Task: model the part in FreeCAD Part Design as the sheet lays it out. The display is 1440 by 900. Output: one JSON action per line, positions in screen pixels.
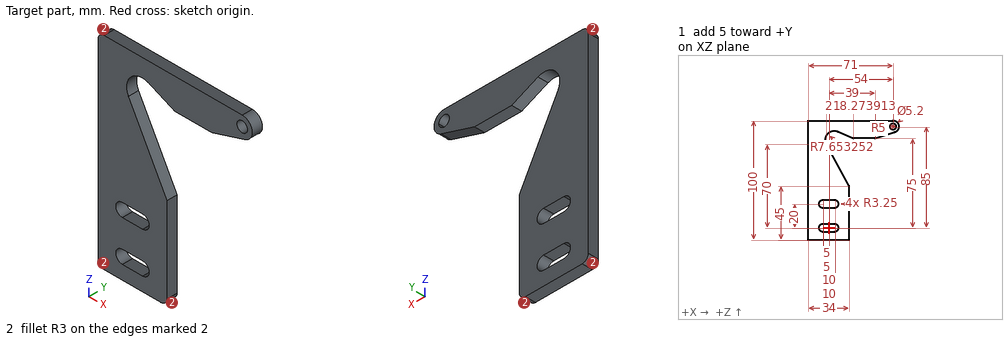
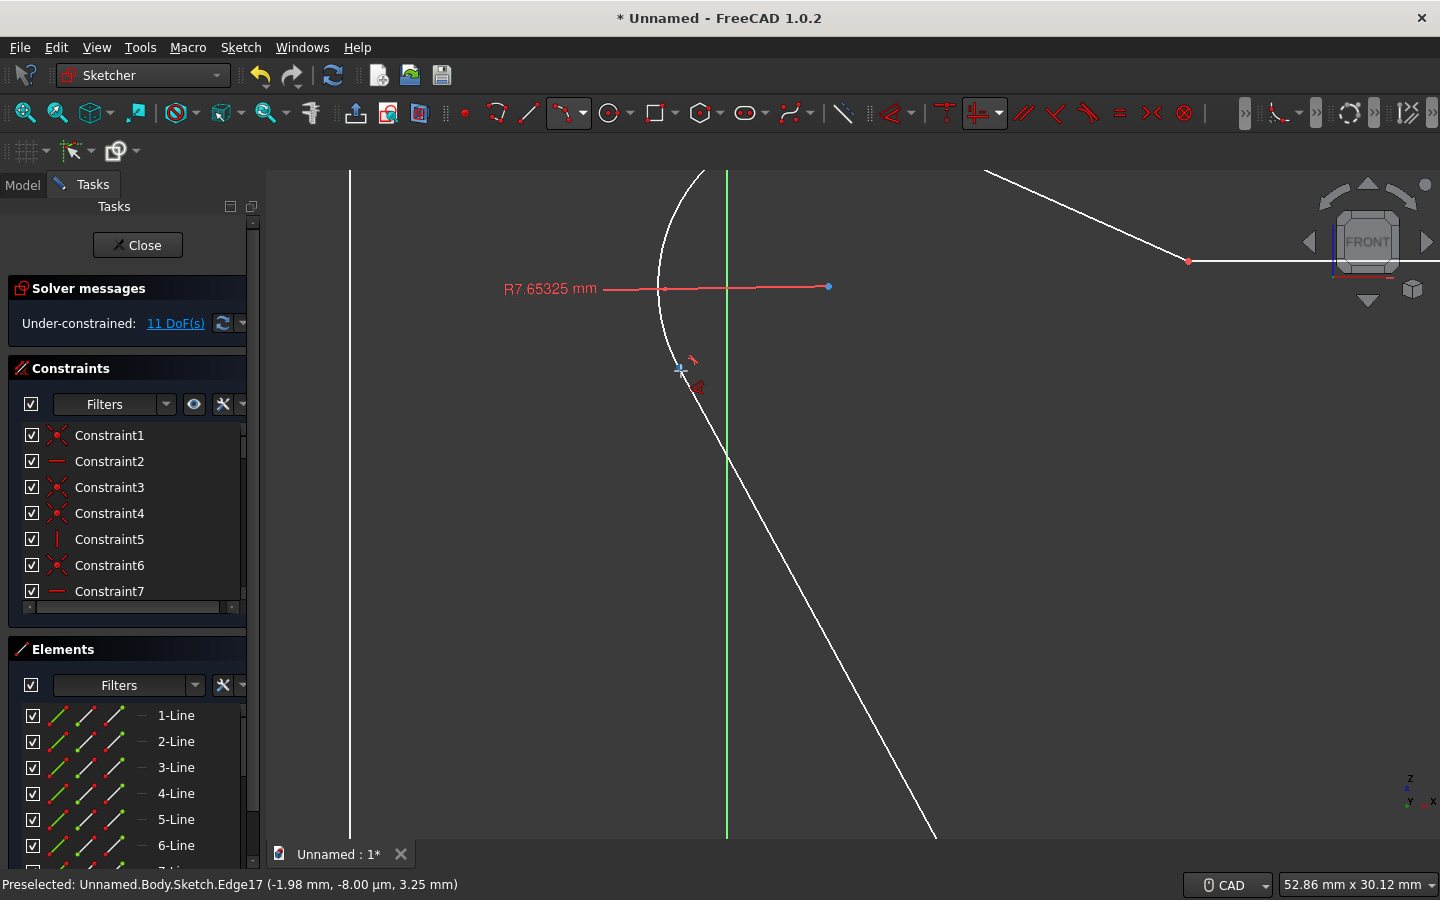
{"action": "left_click", "coordinate": [679, 368]}
{"action": "left_click", "coordinate": [703, 334]}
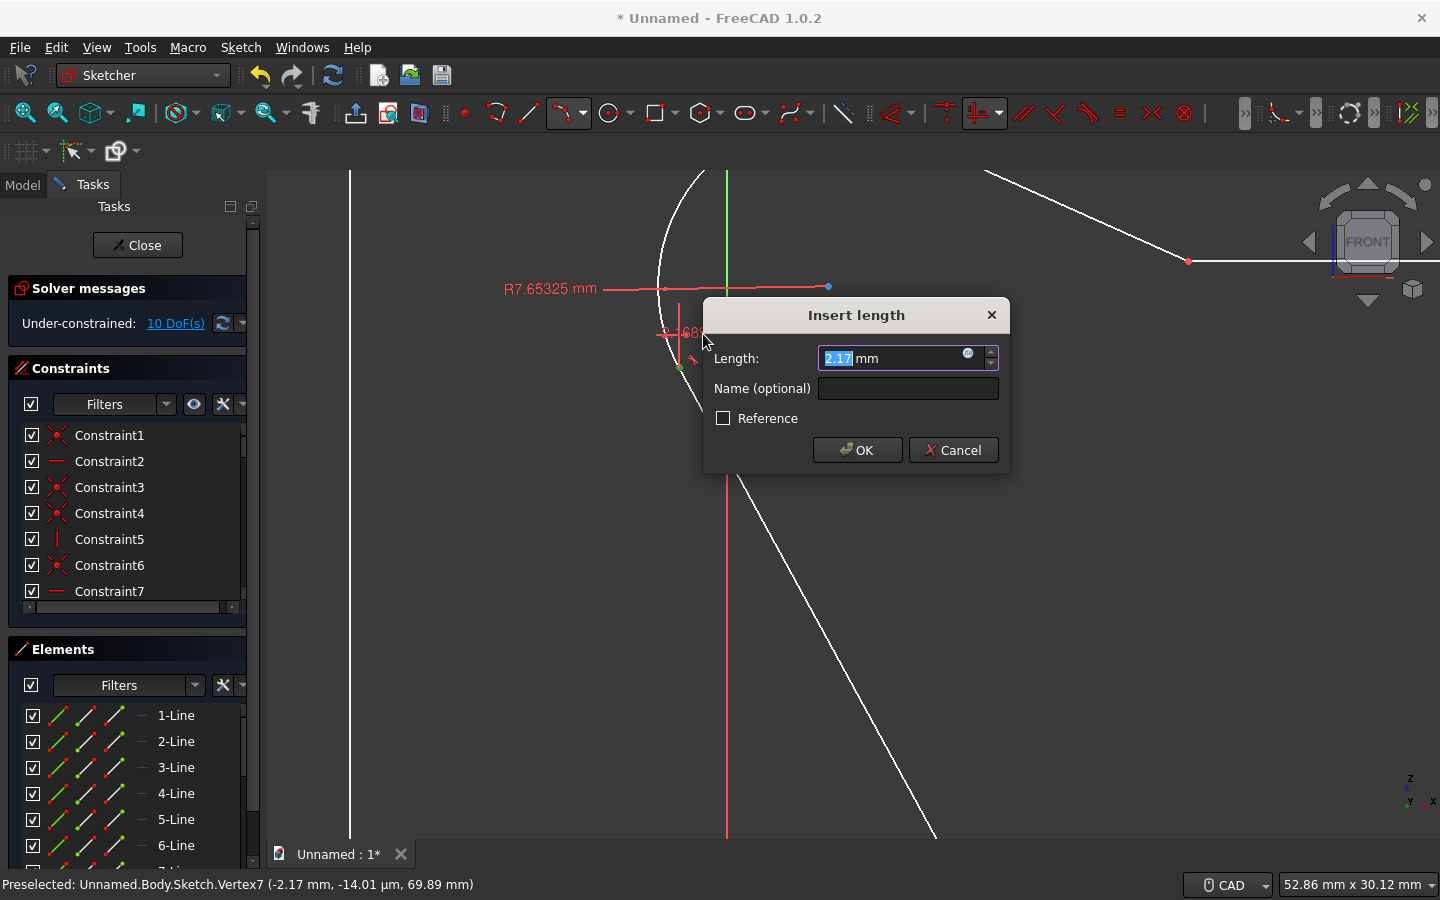
{"action": "type", "text": "2"}
{"action": "key", "text": "Return"}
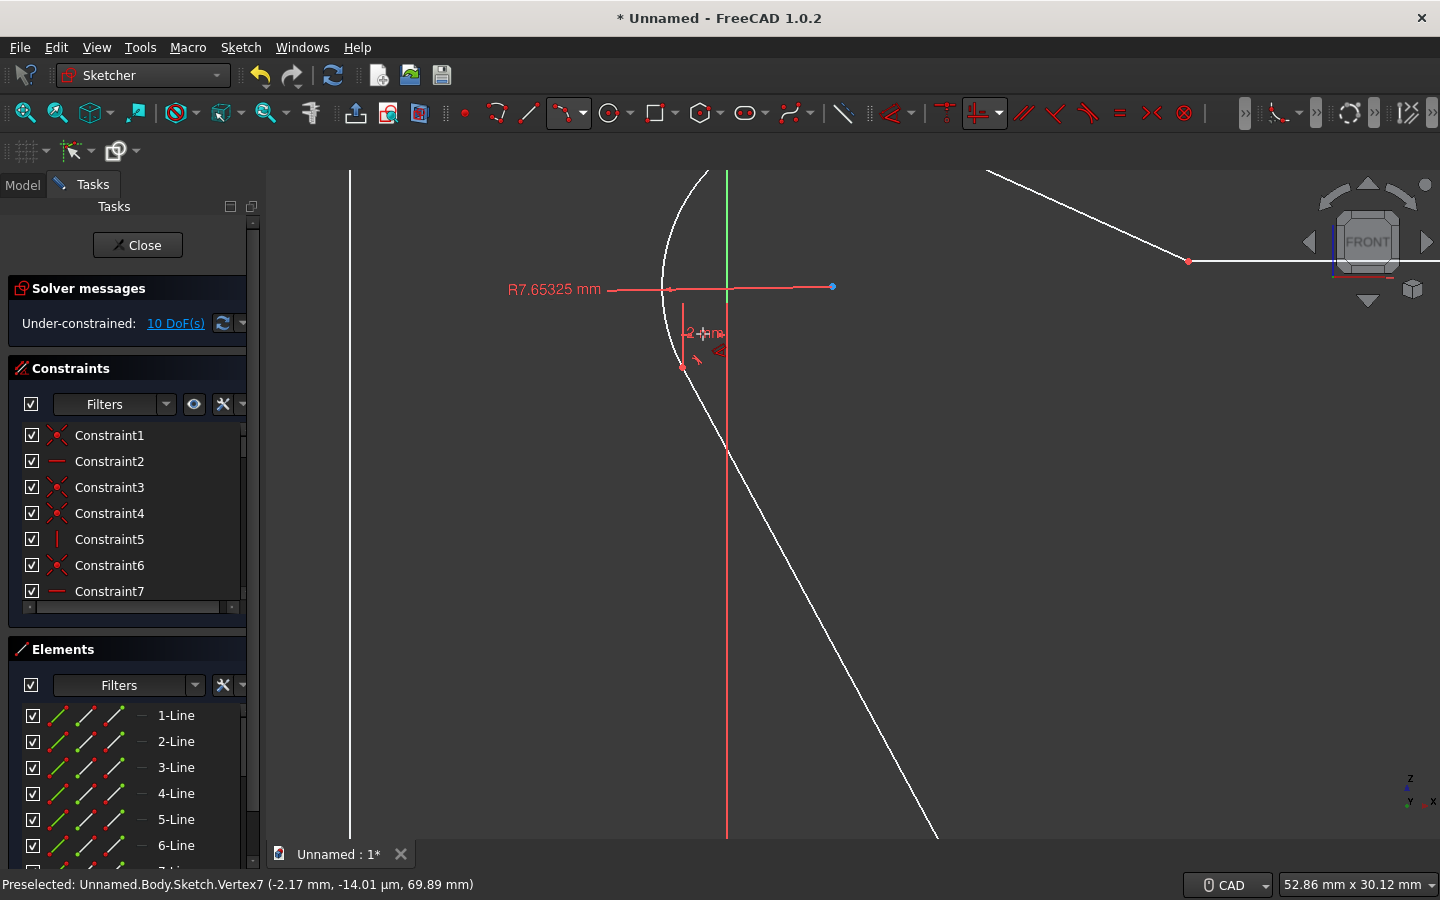
{"action": "scroll", "coordinate": [681, 371], "scroll_direction": "down", "scroll_amount": 8}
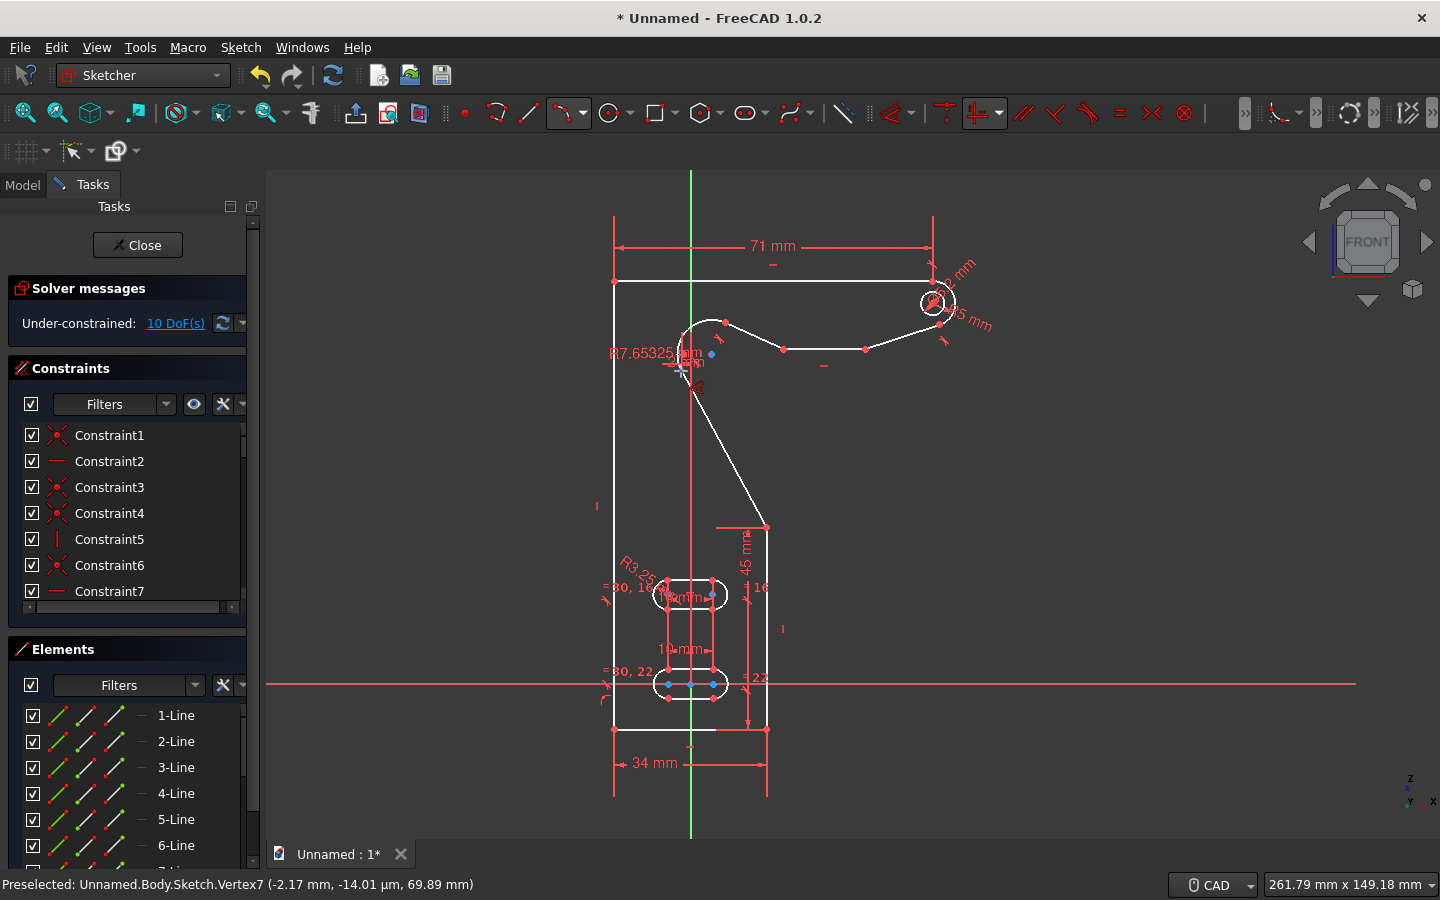
{"action": "scroll", "coordinate": [668, 580], "scroll_direction": "up", "scroll_amount": 3}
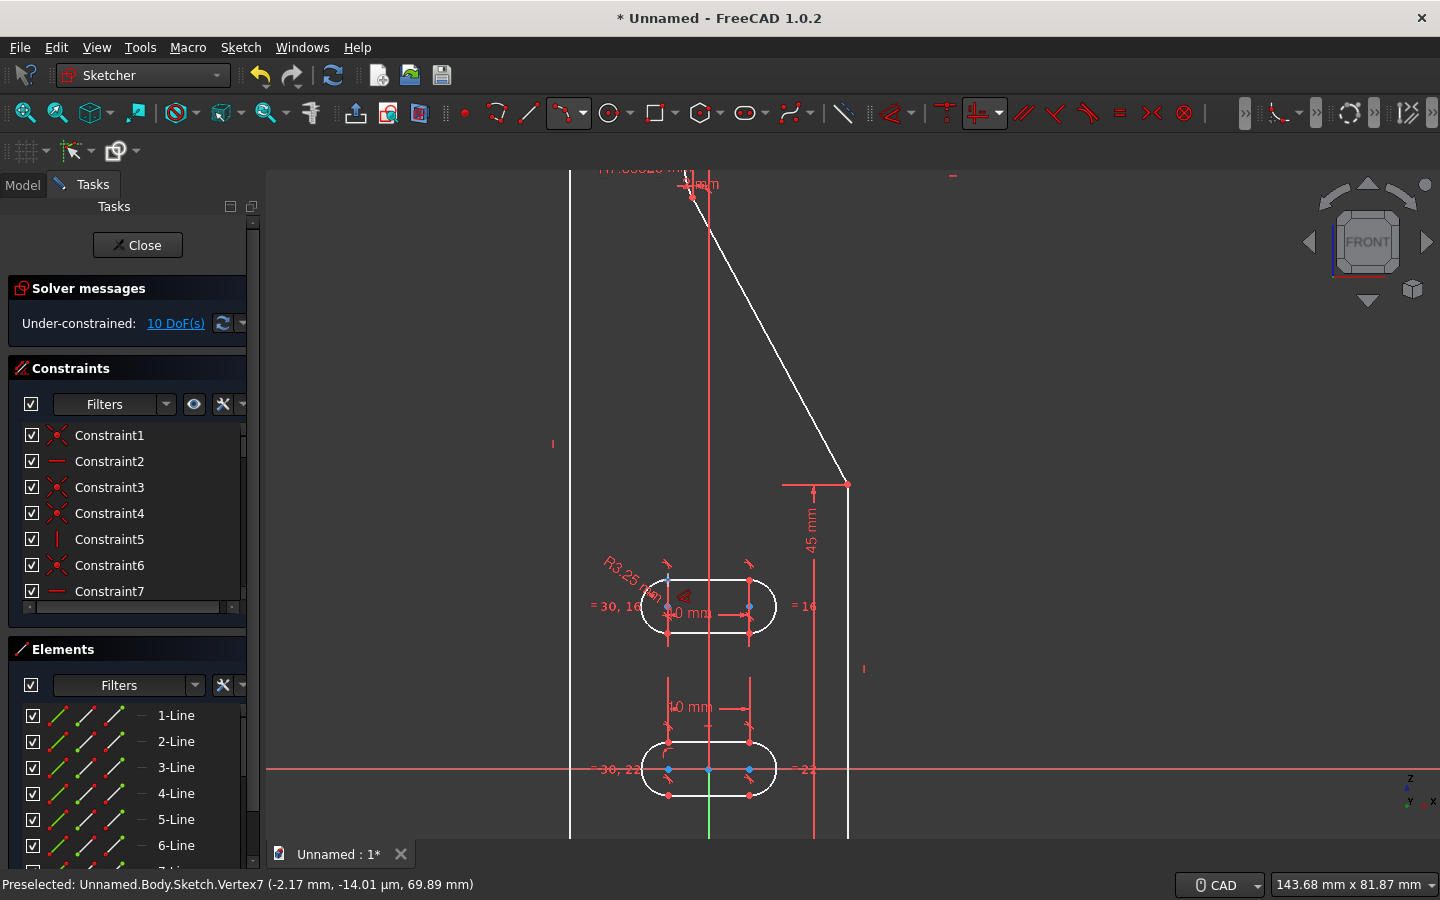
{"action": "left_click", "coordinate": [668, 580]}
{"action": "left_click", "coordinate": [688, 546]}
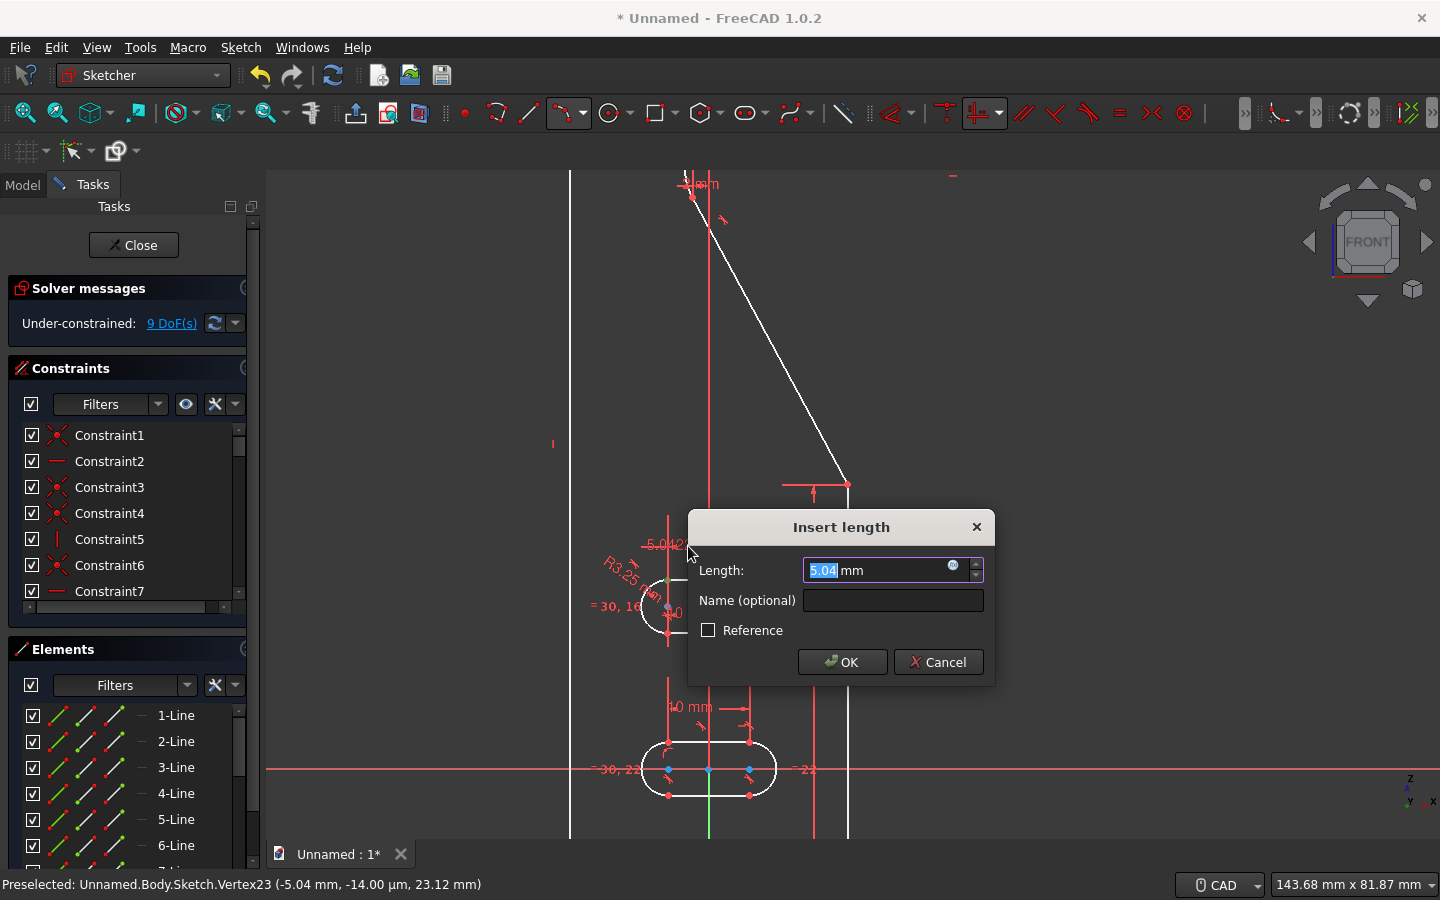
{"action": "type", "text": "5"}
{"action": "key", "text": "Return"}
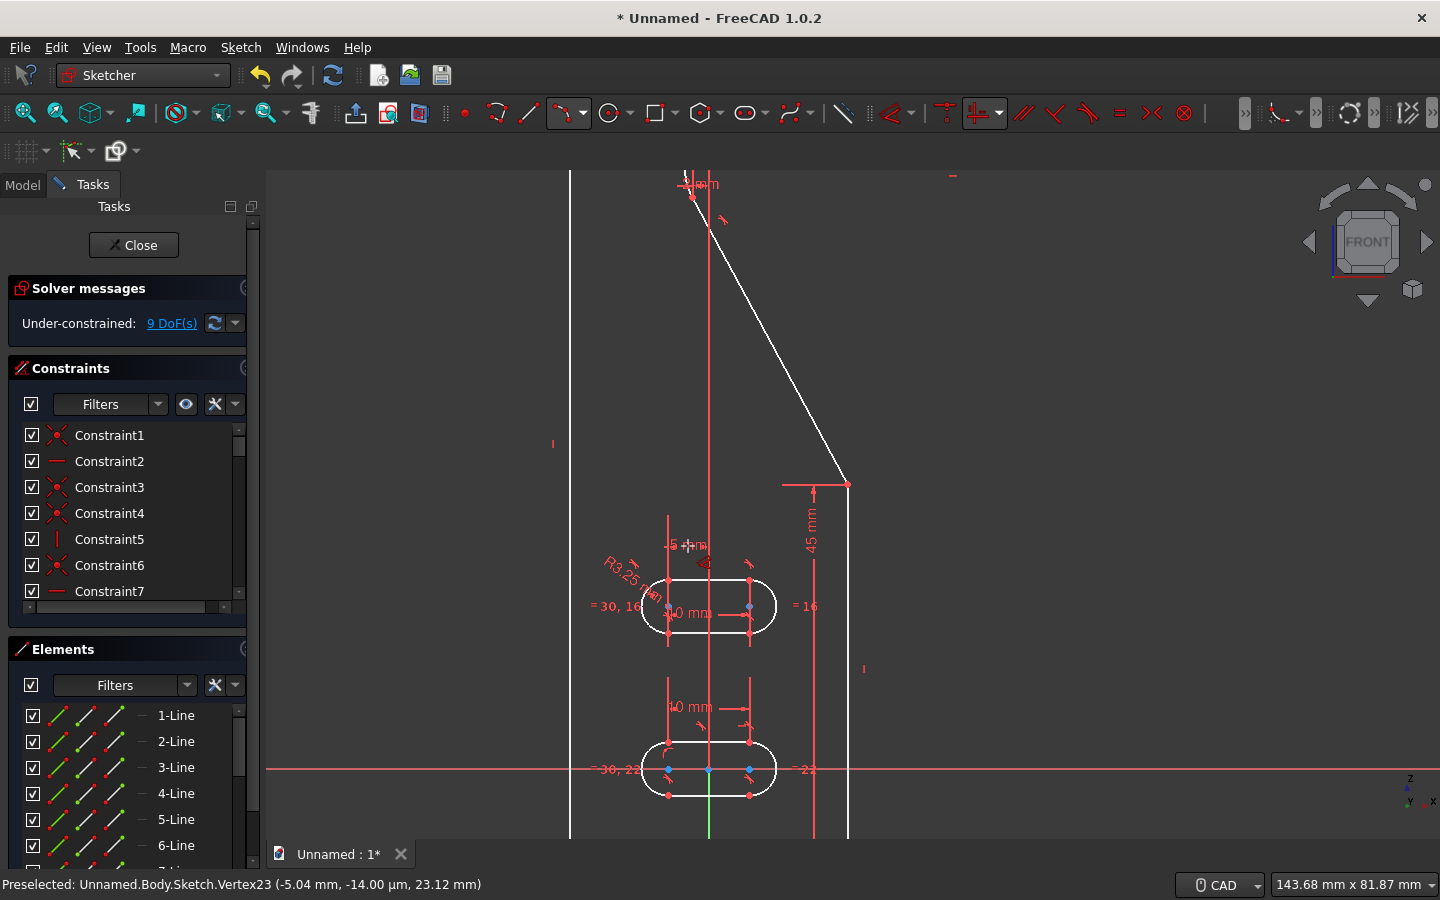
{"action": "left_click", "coordinate": [668, 742]}
{"action": "left_click", "coordinate": [688, 684]}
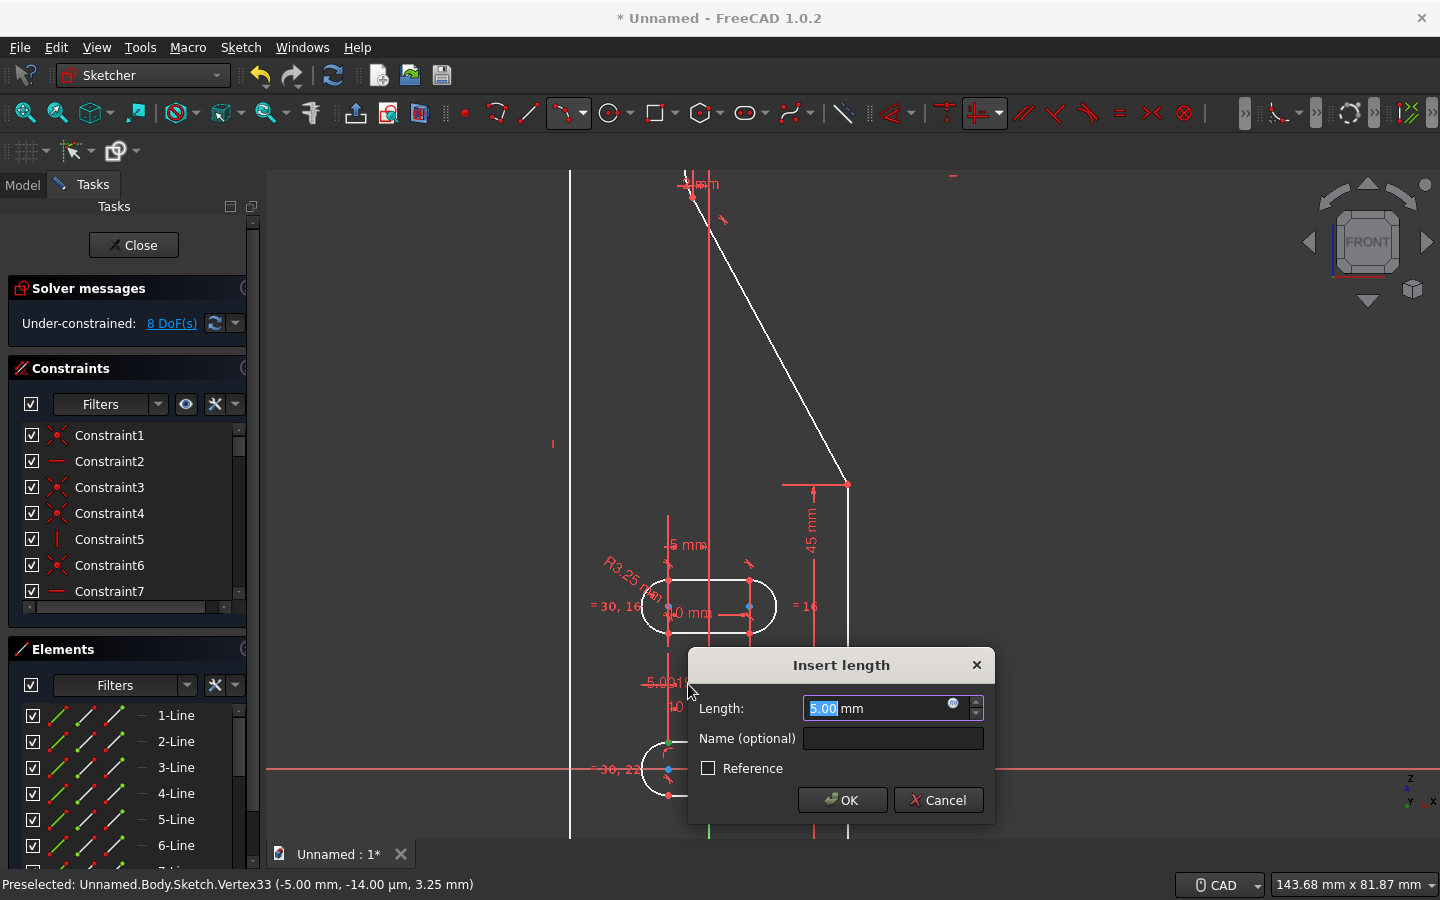
{"action": "type", "text": "5"}
{"action": "key", "text": "Return"}